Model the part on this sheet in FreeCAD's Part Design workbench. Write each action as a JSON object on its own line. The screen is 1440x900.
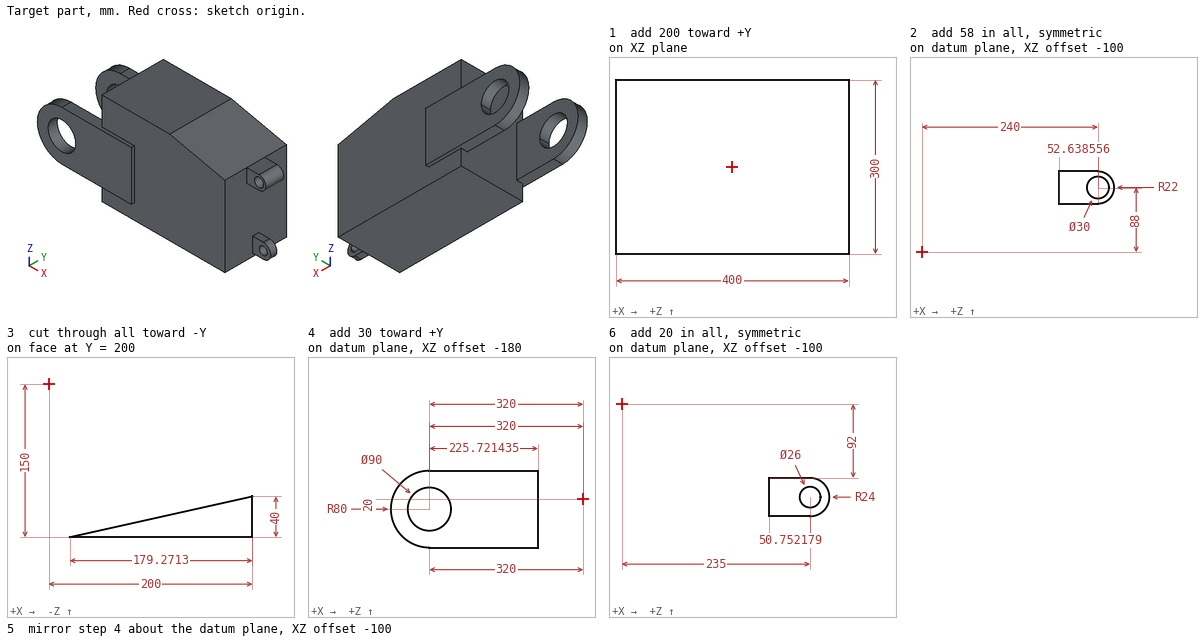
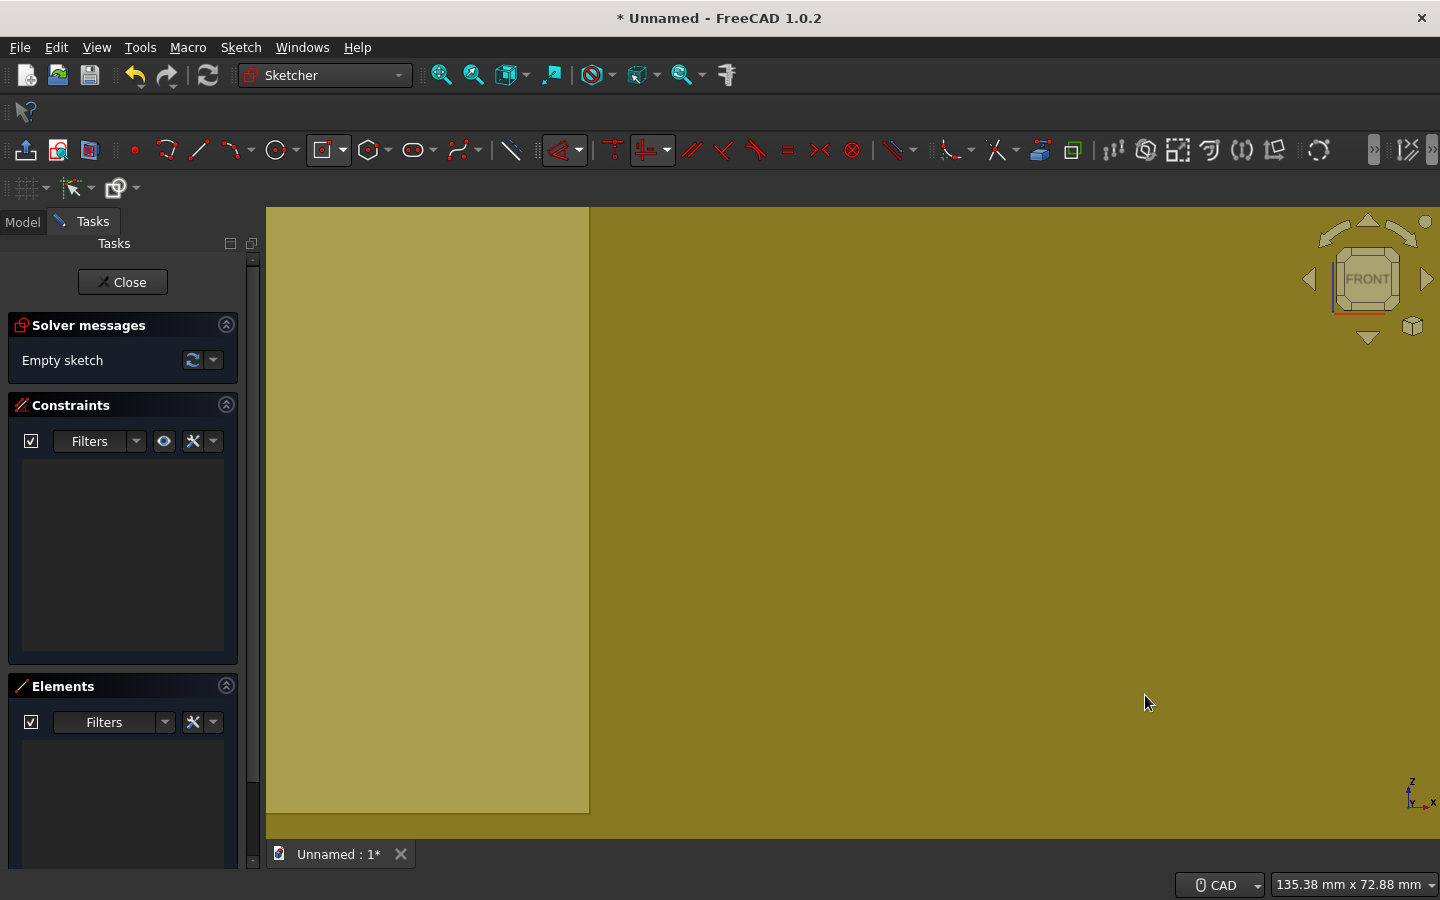
{"action": "left_click", "coordinate": [168, 150]}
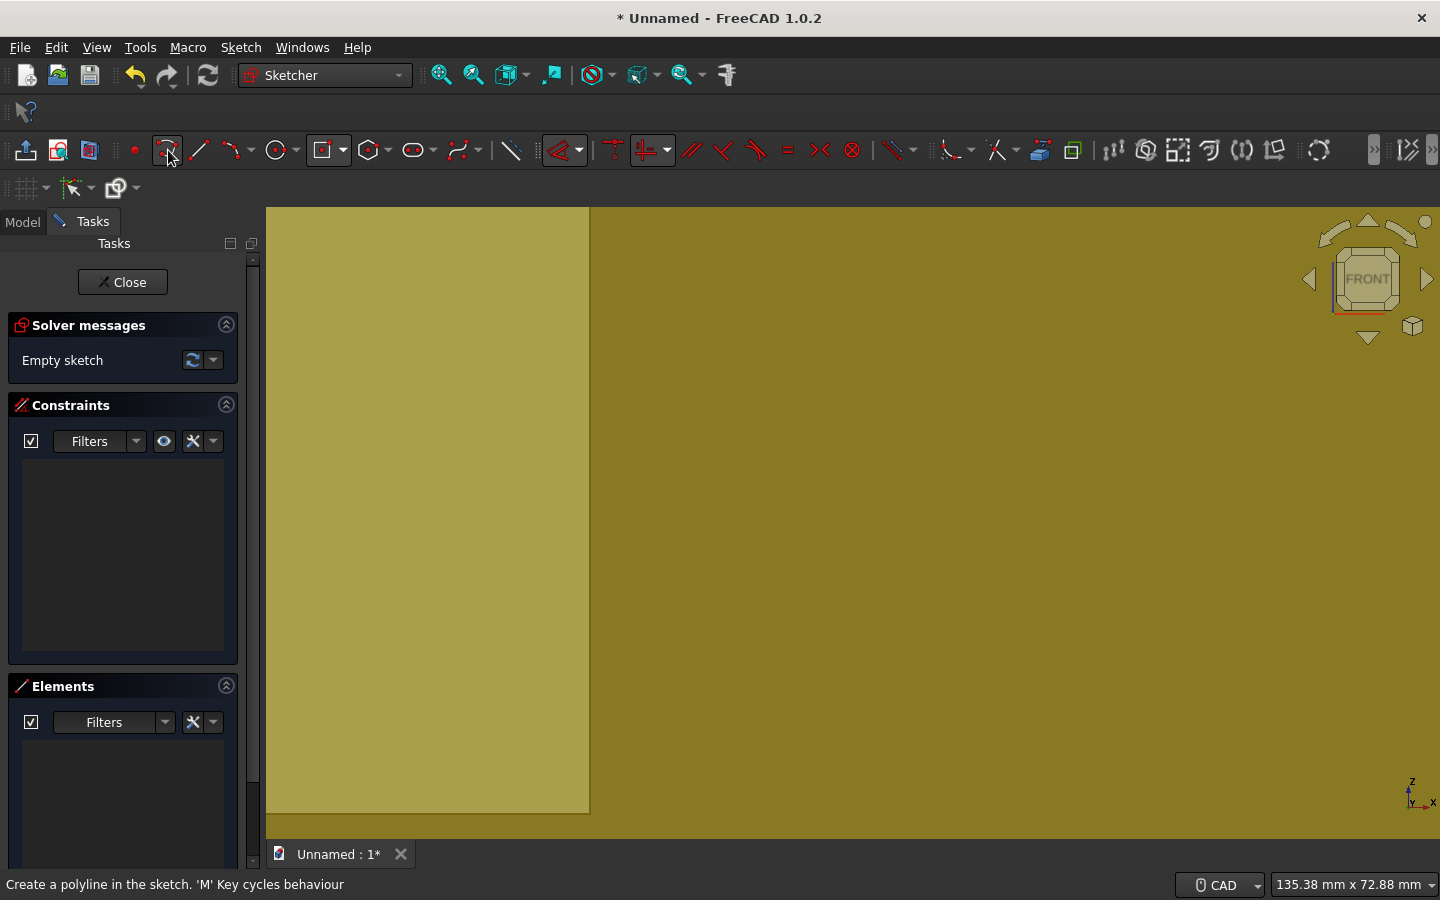
{"action": "left_click", "coordinate": [894, 727]}
{"action": "left_click", "coordinate": [454, 727]}
{"action": "left_click", "coordinate": [454, 311]}
{"action": "left_click", "coordinate": [894, 311]}
{"action": "right_click", "coordinate": [894, 311]}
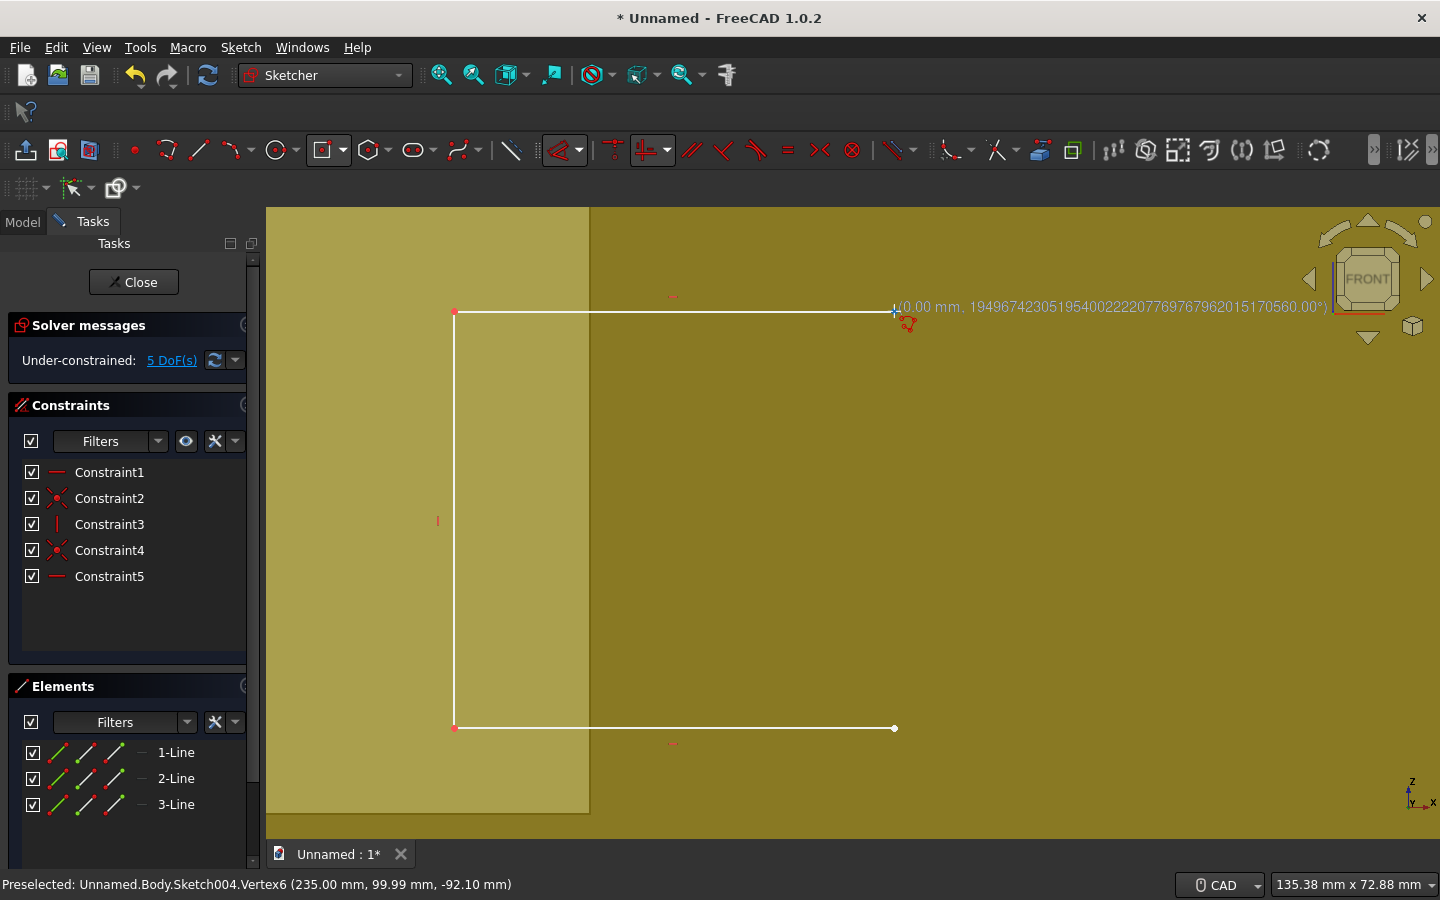
{"action": "left_click", "coordinate": [232, 150]}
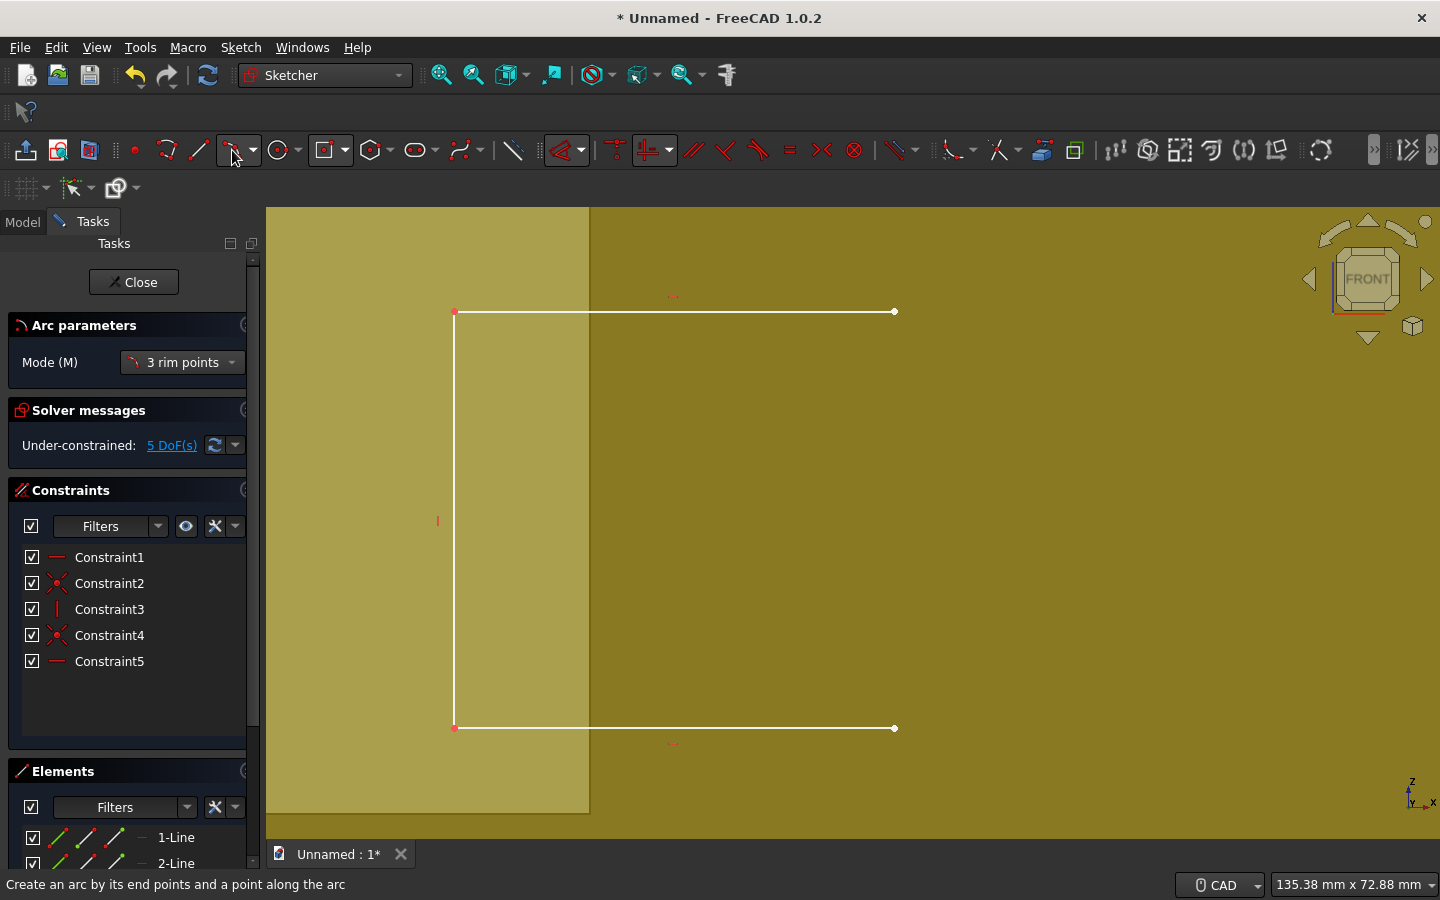
{"action": "left_click", "coordinate": [894, 312]}
{"action": "left_click", "coordinate": [894, 728]}
{"action": "left_click", "coordinate": [1102, 519]}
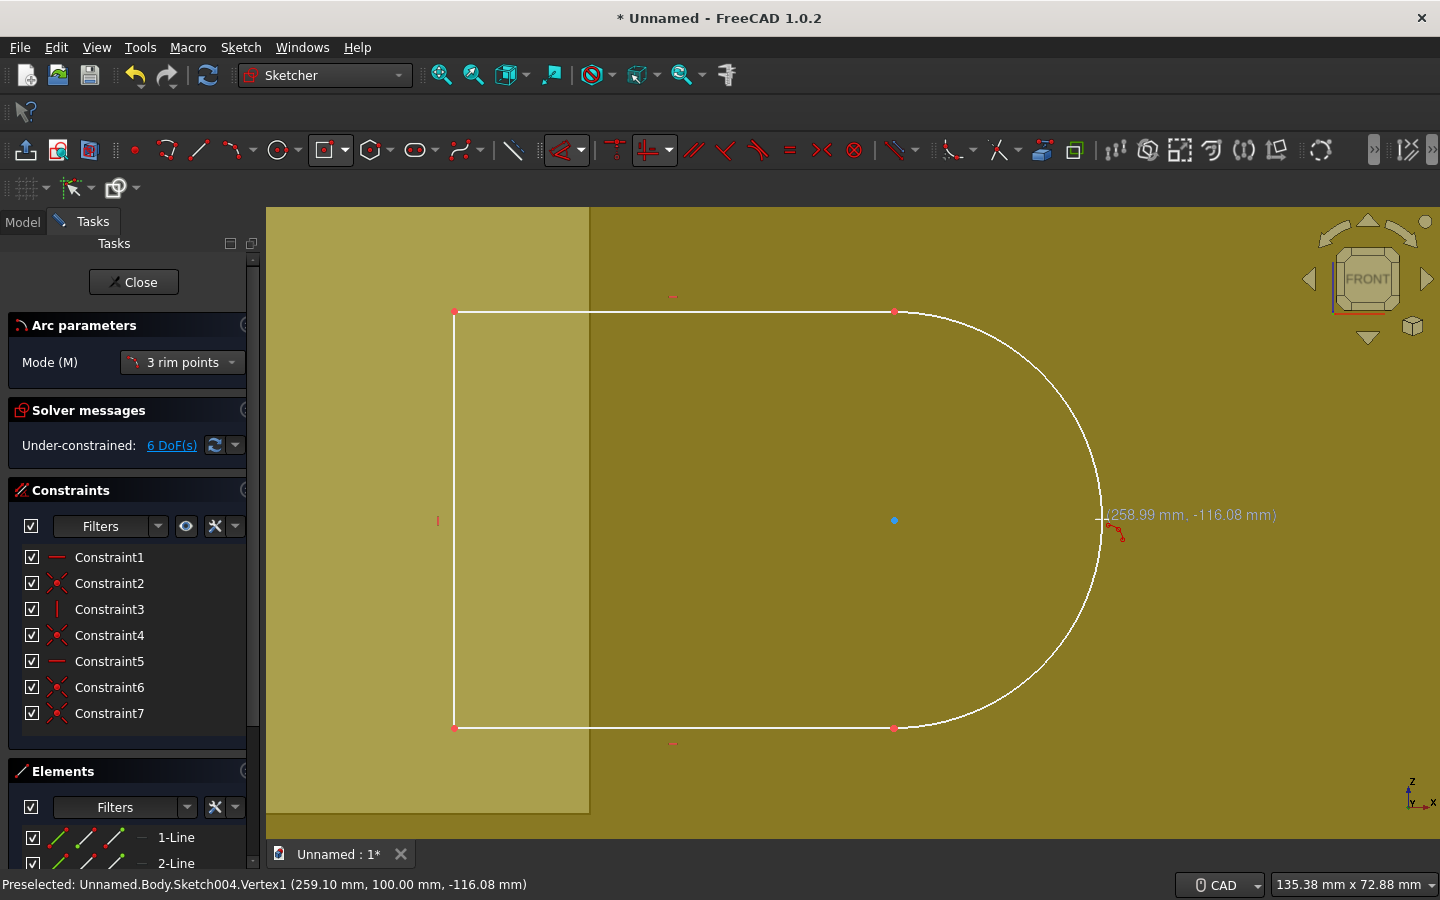
{"action": "left_click", "coordinate": [278, 150]}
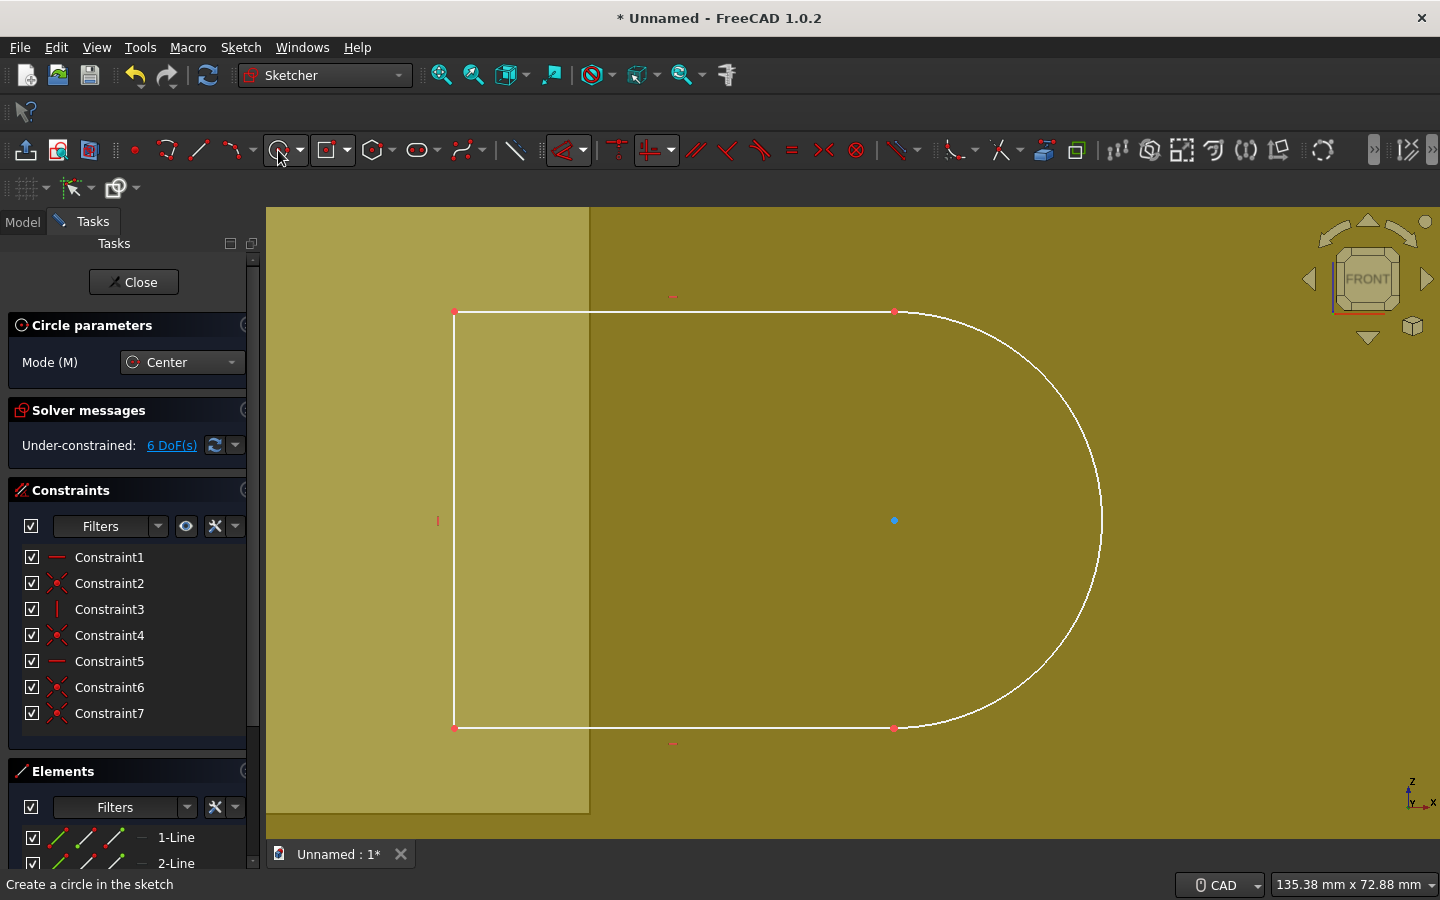
{"action": "left_click", "coordinate": [894, 519]}
{"action": "left_click", "coordinate": [974, 440]}
{"action": "key", "text": "Escape"}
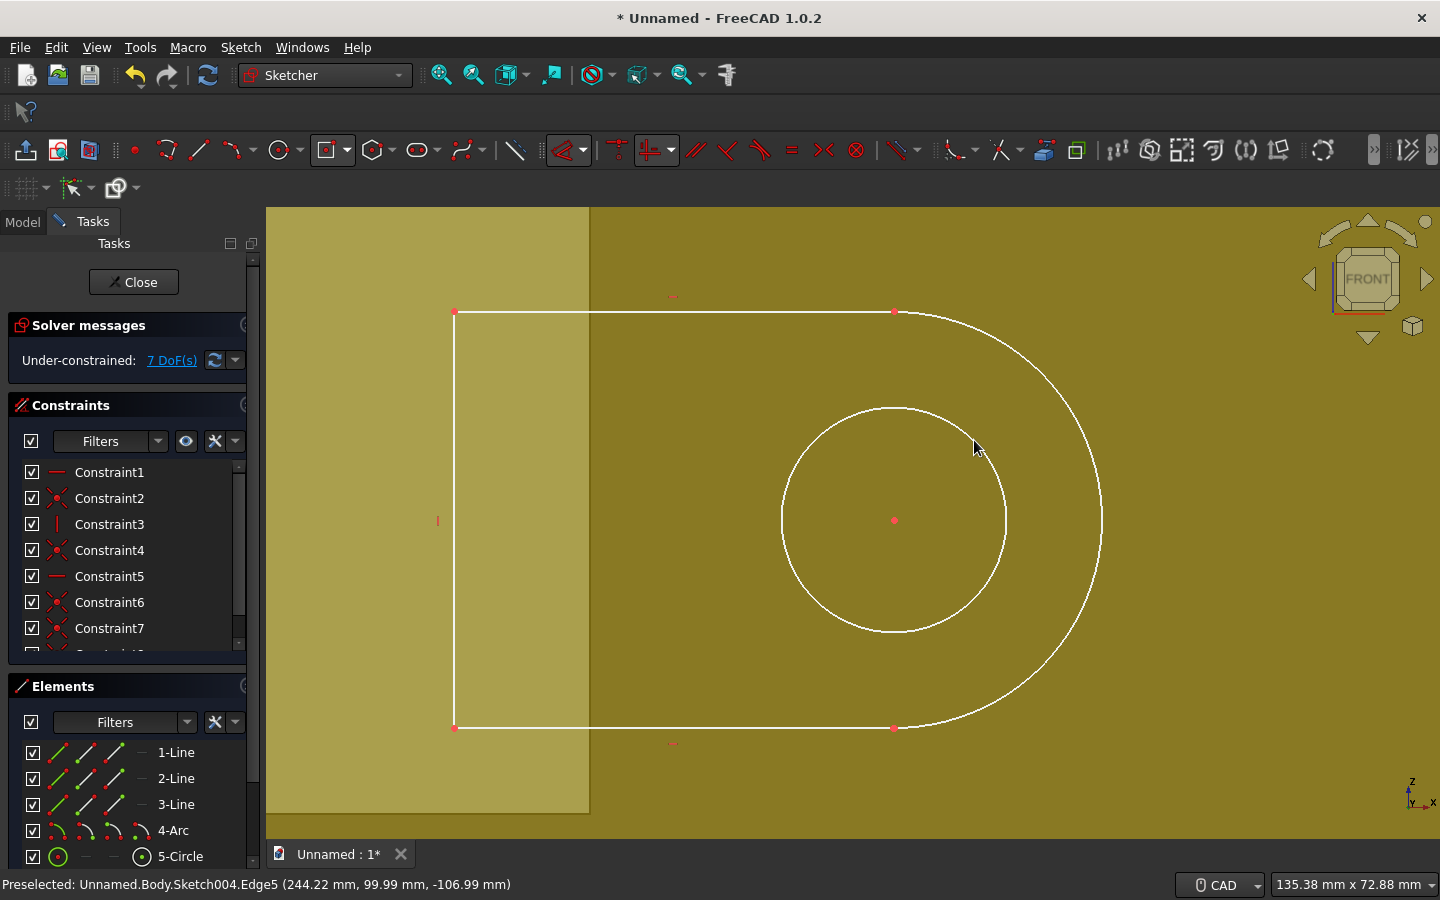
{"action": "left_click", "coordinate": [762, 728]}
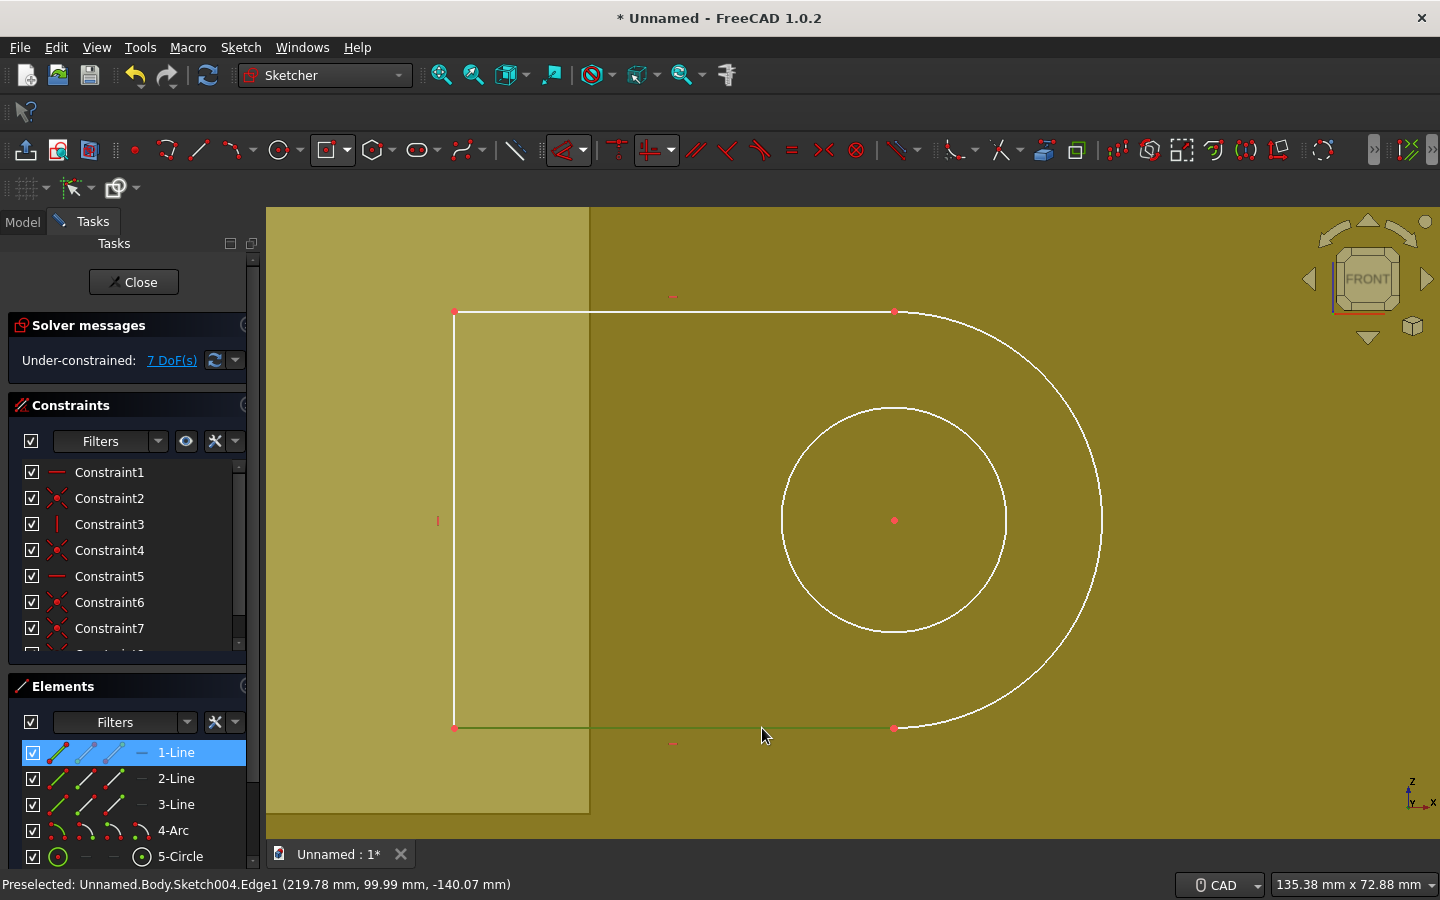
{"action": "left_click", "coordinate": [1062, 642]}